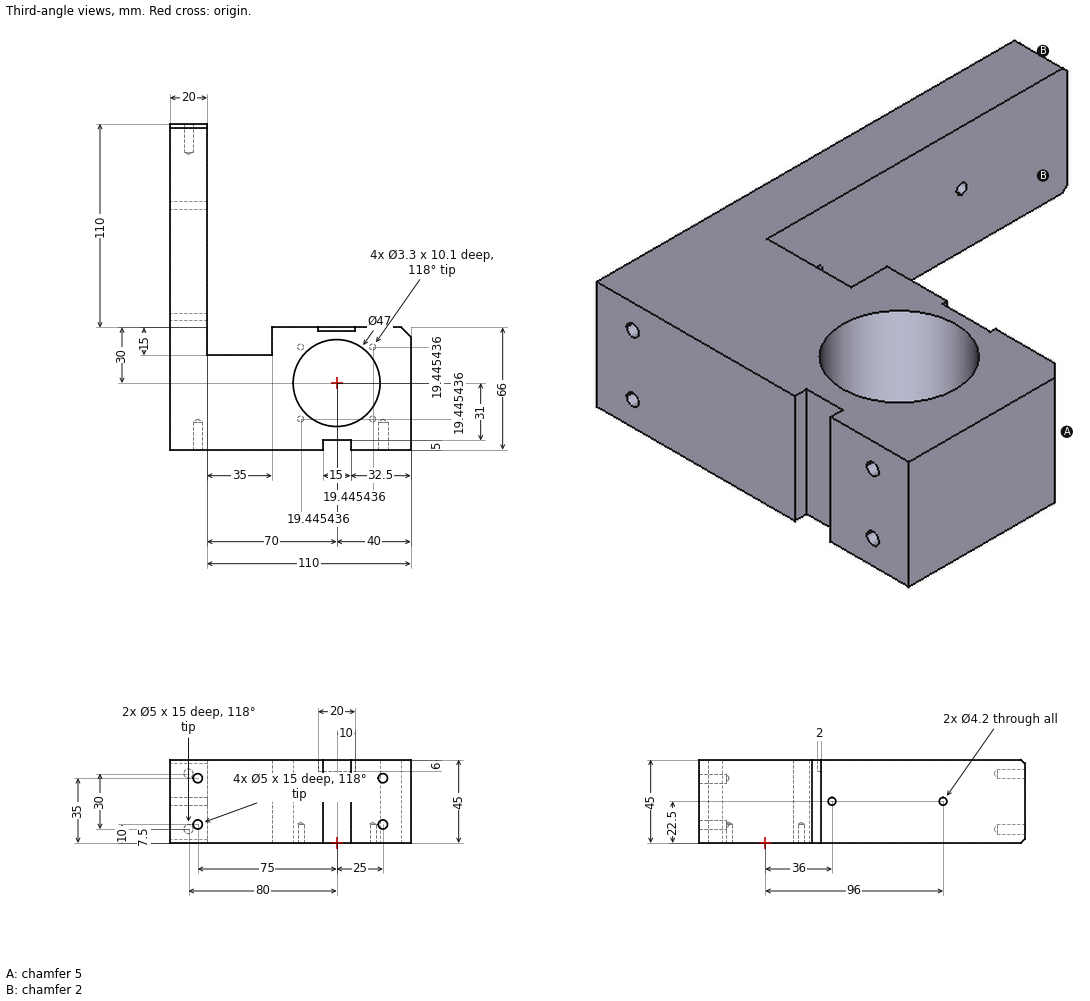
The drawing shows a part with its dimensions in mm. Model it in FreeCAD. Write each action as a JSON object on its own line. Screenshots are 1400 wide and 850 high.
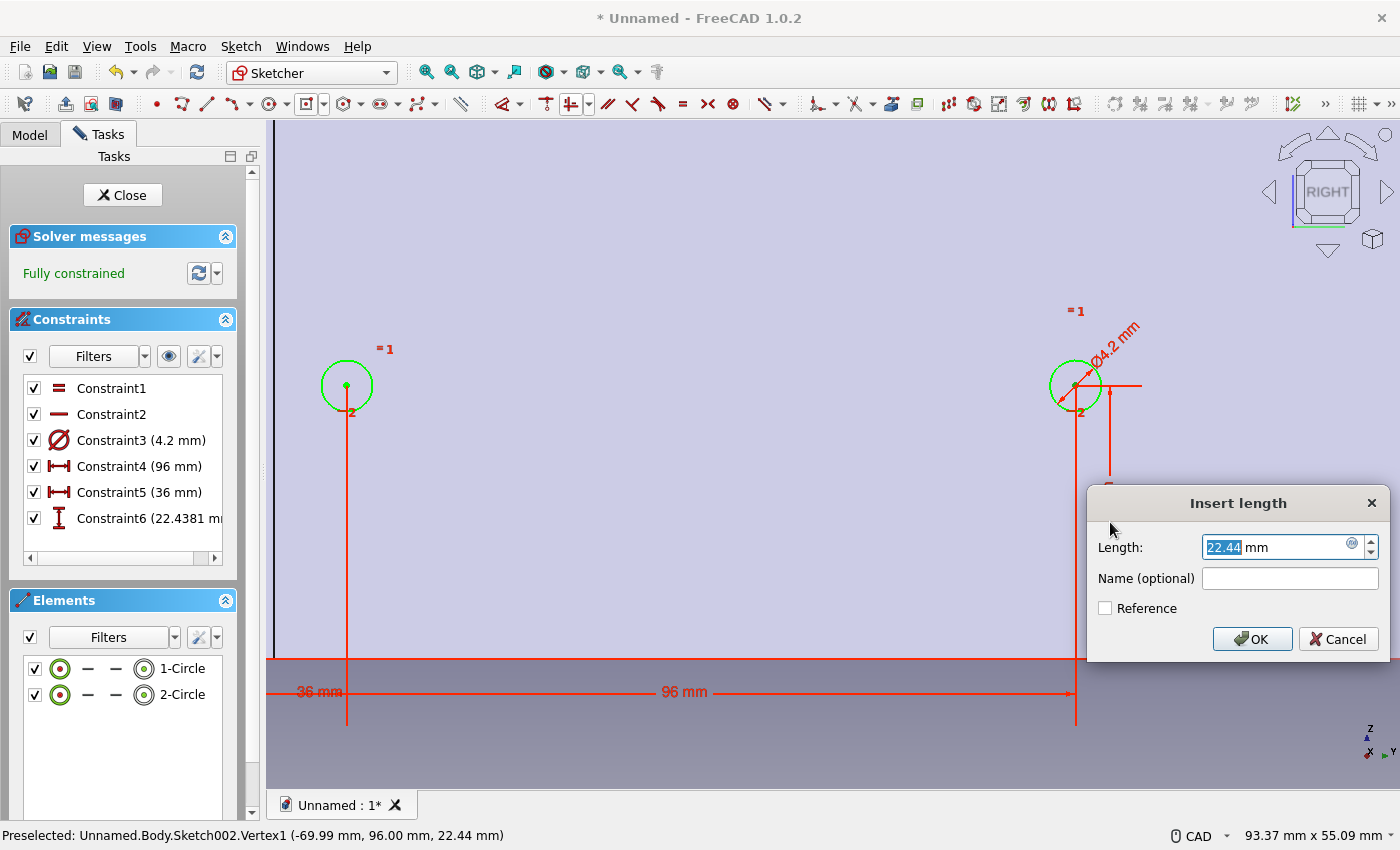
{"action": "type", "text": "22.5"}
{"action": "key", "text": "Return"}
{"action": "key", "text": "Escape"}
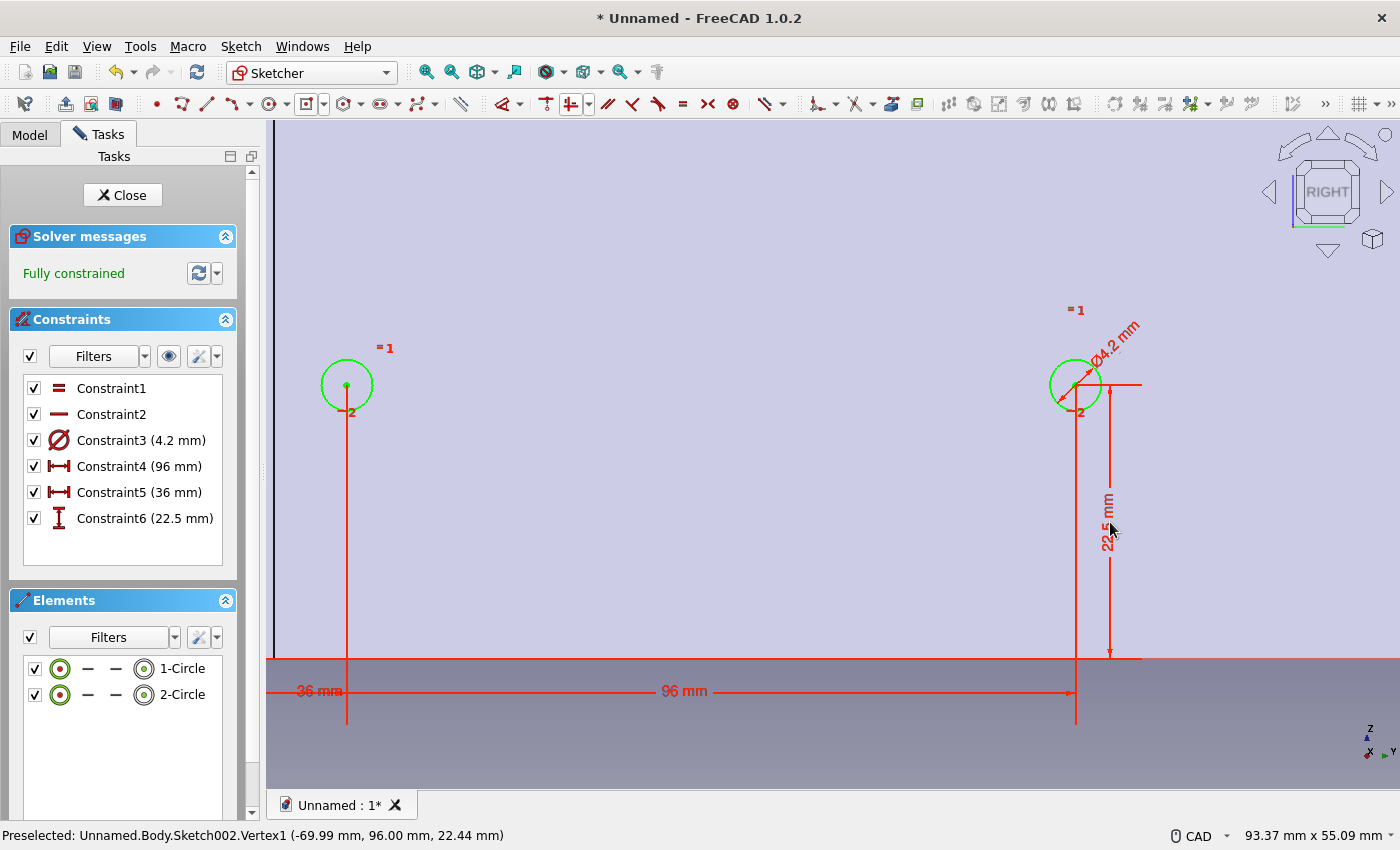
{"action": "left_click", "coordinate": [123, 195]}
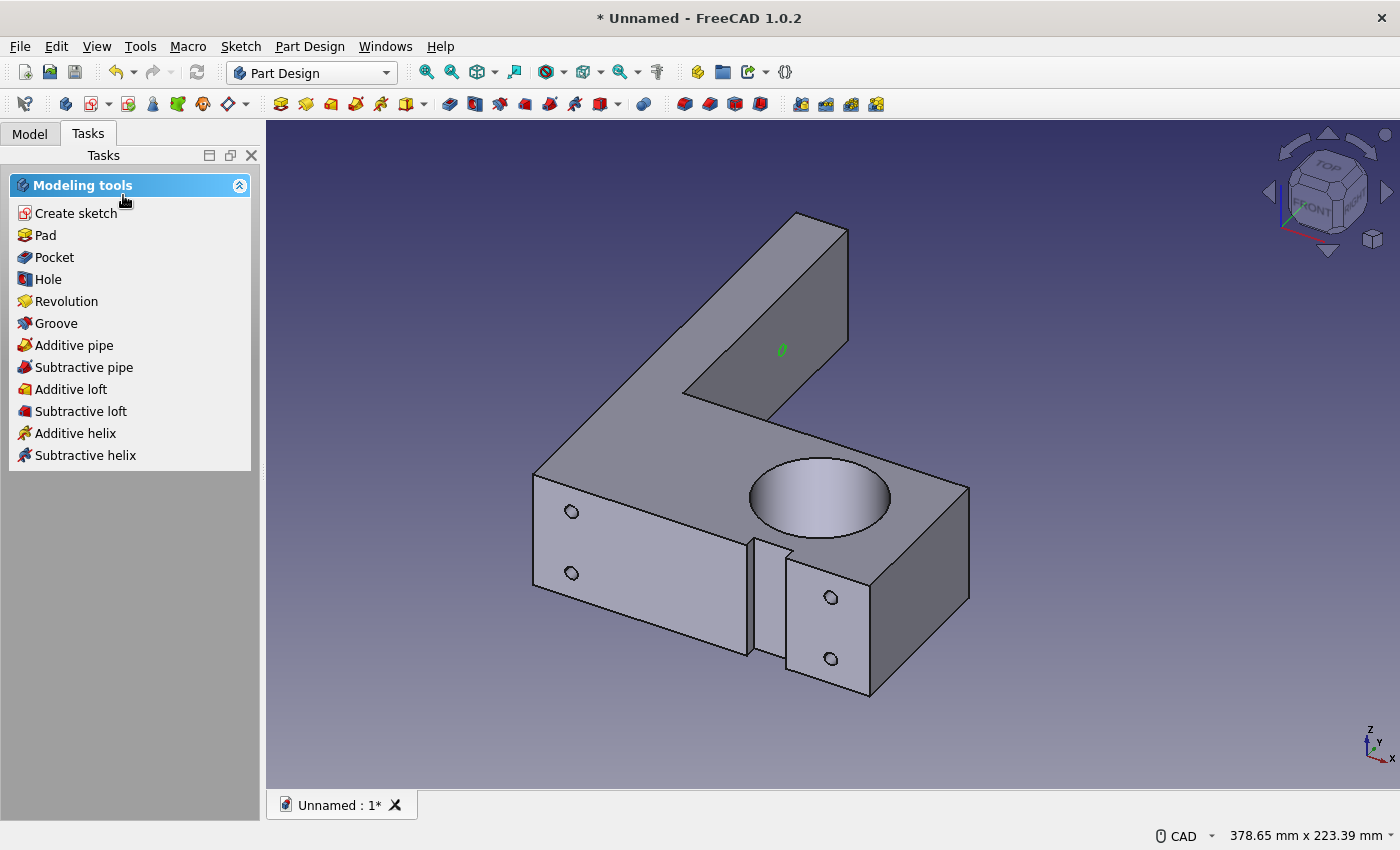
{"action": "left_click", "coordinate": [475, 104]}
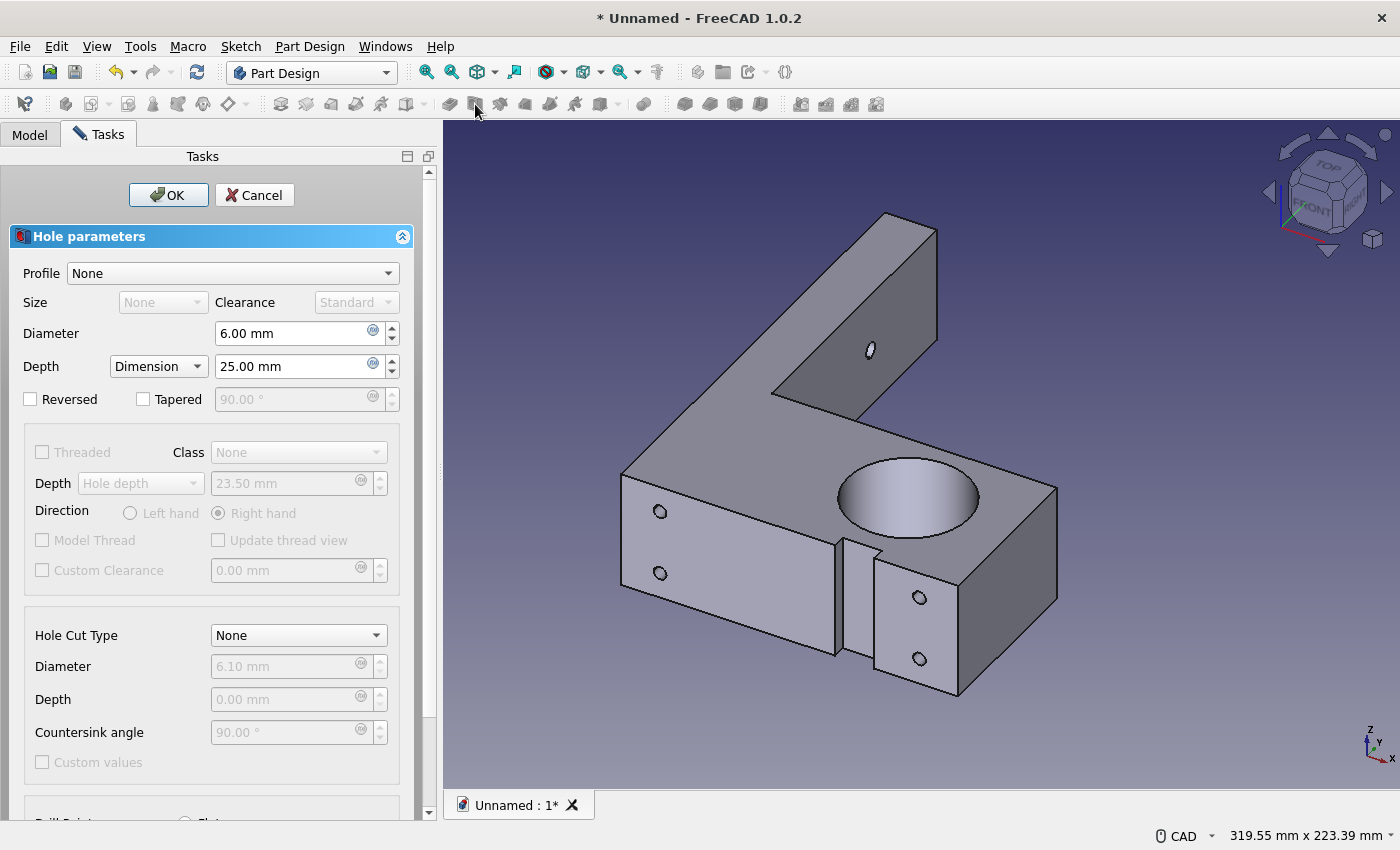
{"action": "triple_click", "coordinate": [300, 334]}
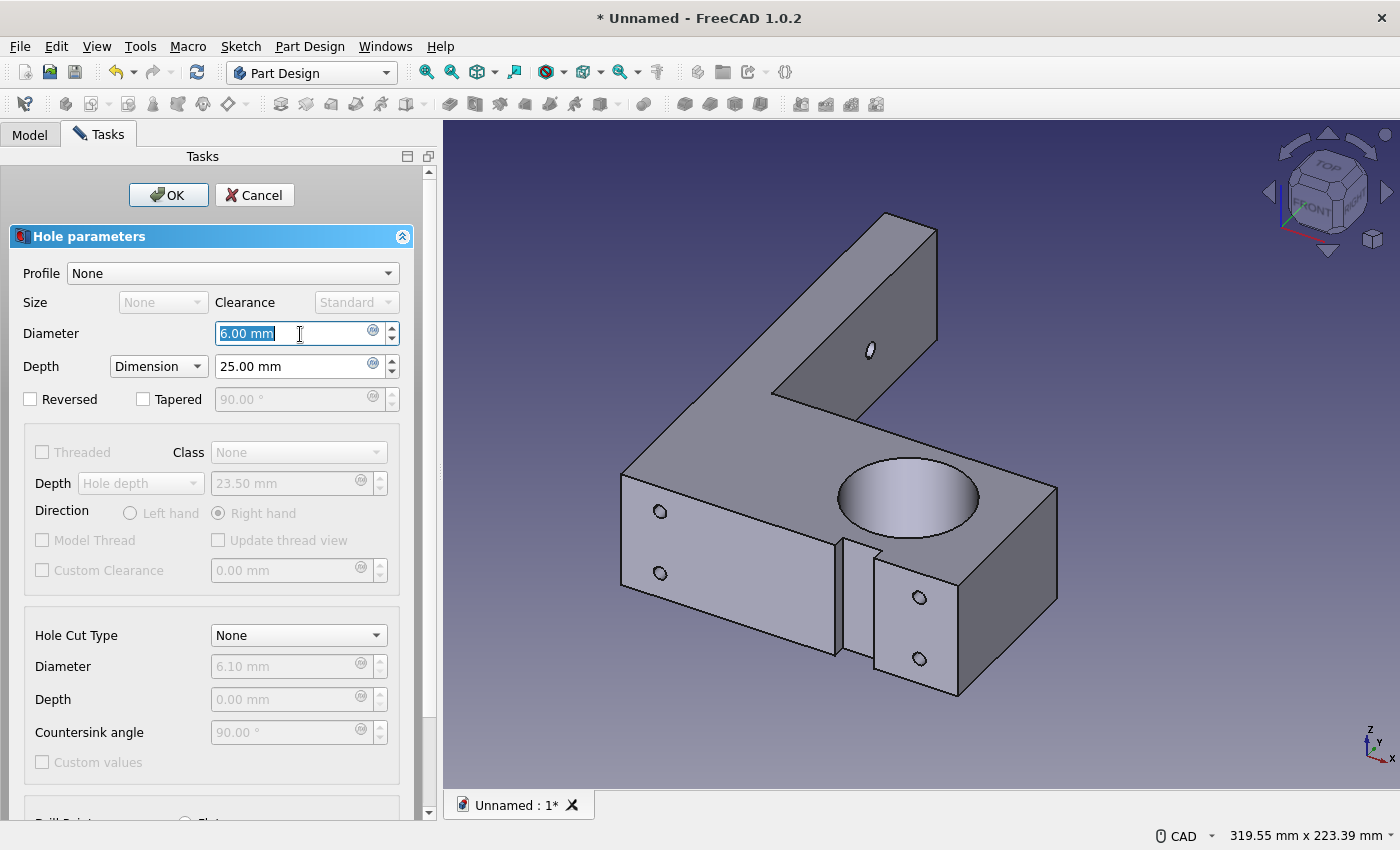
{"action": "type", "text": "4.2"}
{"action": "key", "text": "Tab"}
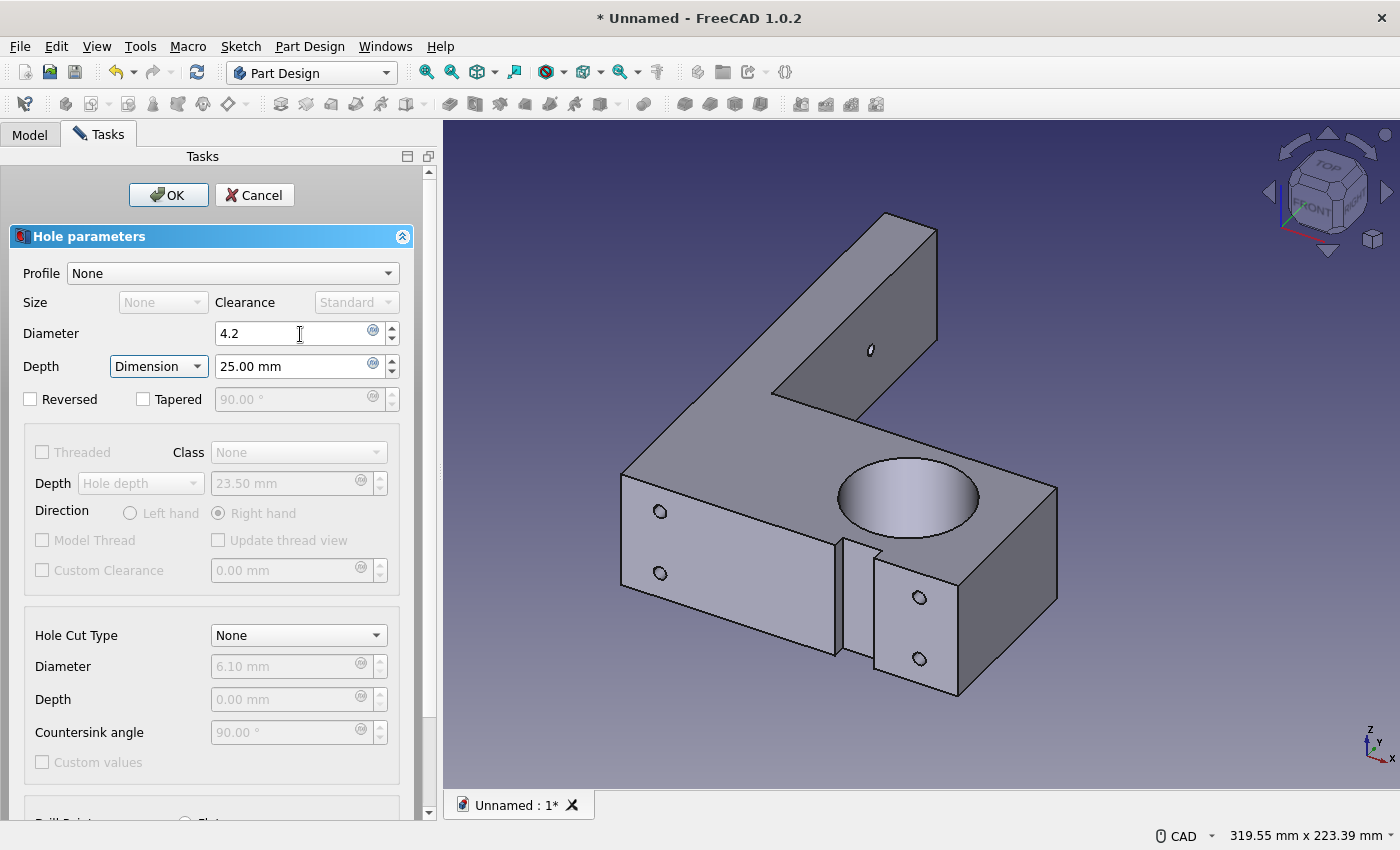
{"action": "left_click", "coordinate": [160, 366]}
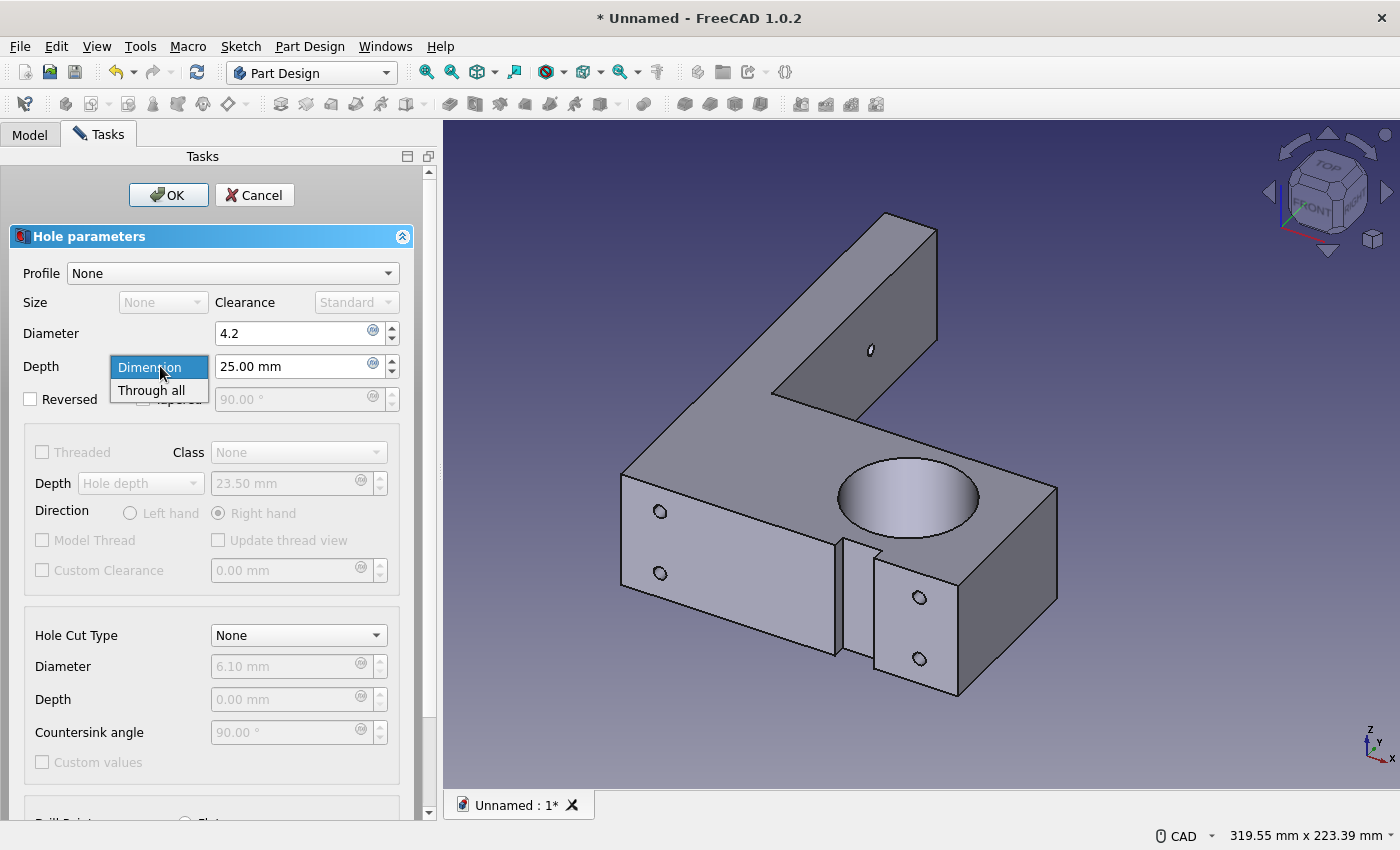
{"action": "left_click", "coordinate": [158, 390]}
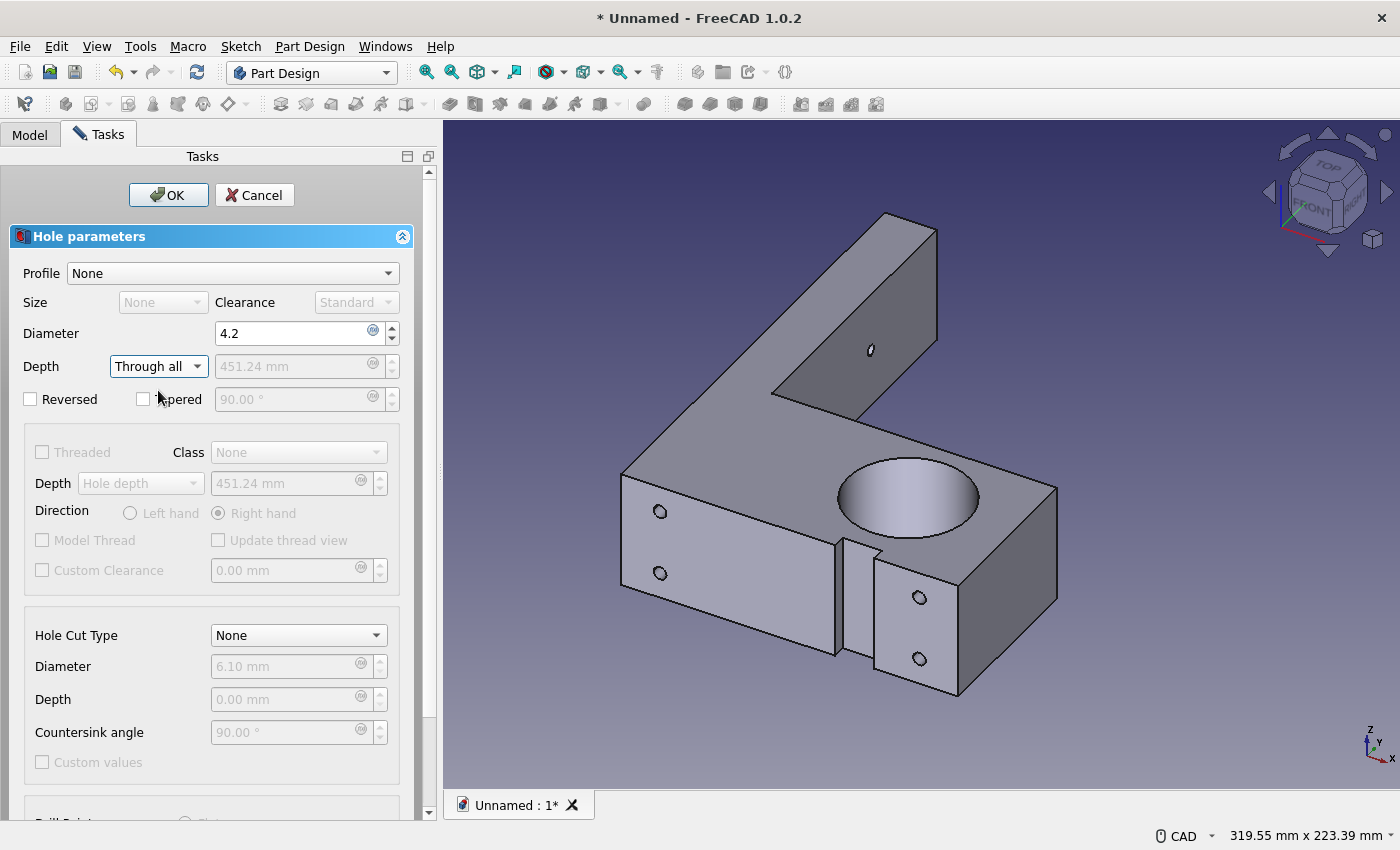
{"action": "left_click", "coordinate": [169, 195]}